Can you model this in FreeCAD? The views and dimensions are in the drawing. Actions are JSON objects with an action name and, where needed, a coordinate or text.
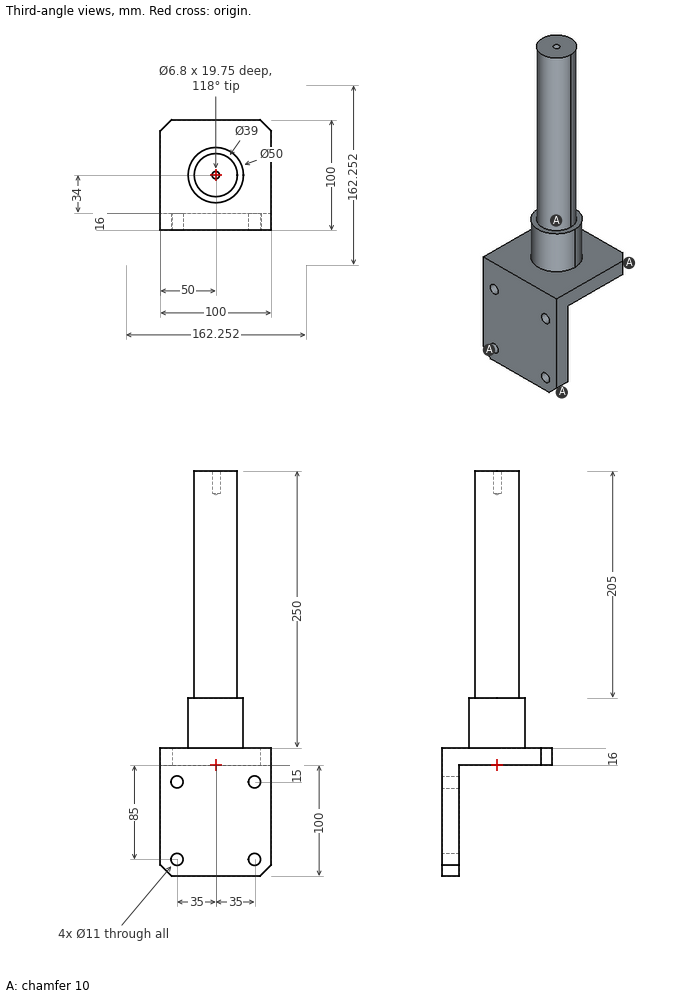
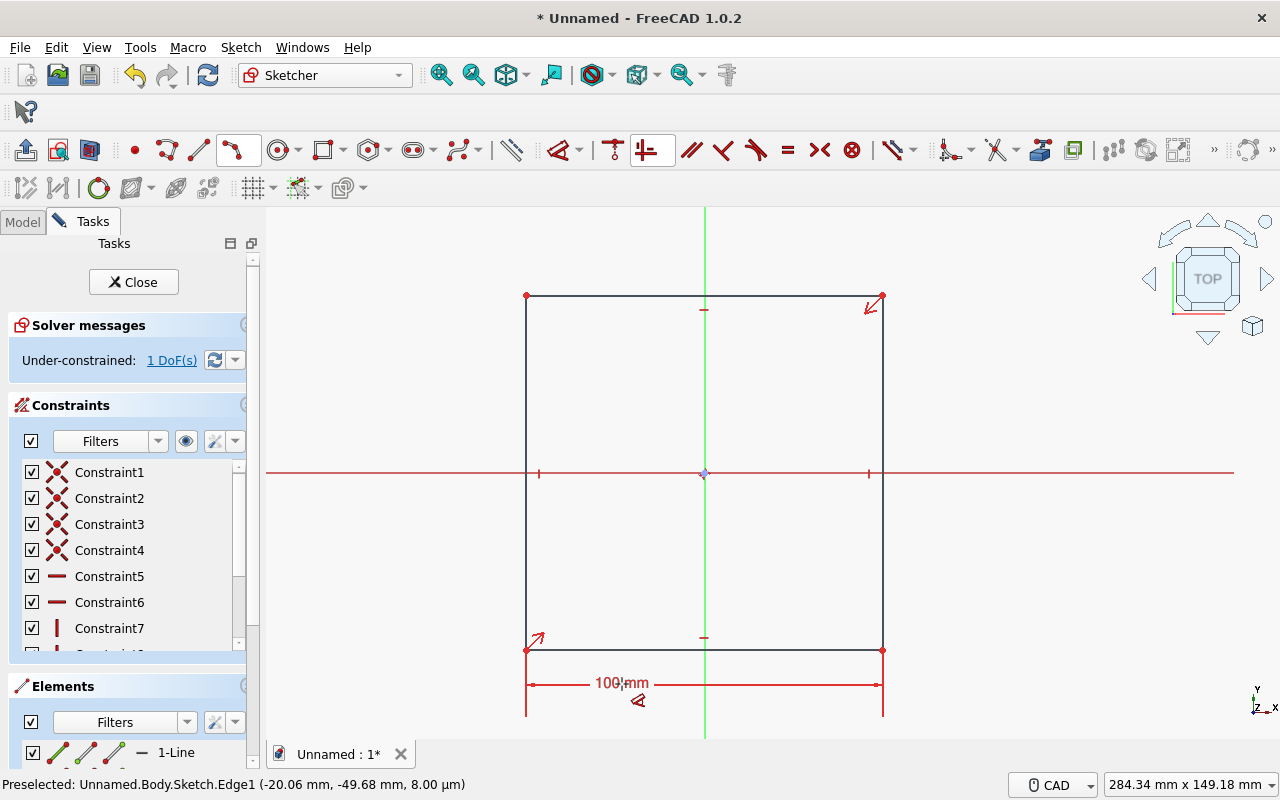
{"action": "left_click", "coordinate": [883, 544]}
{"action": "left_click", "coordinate": [917, 392]}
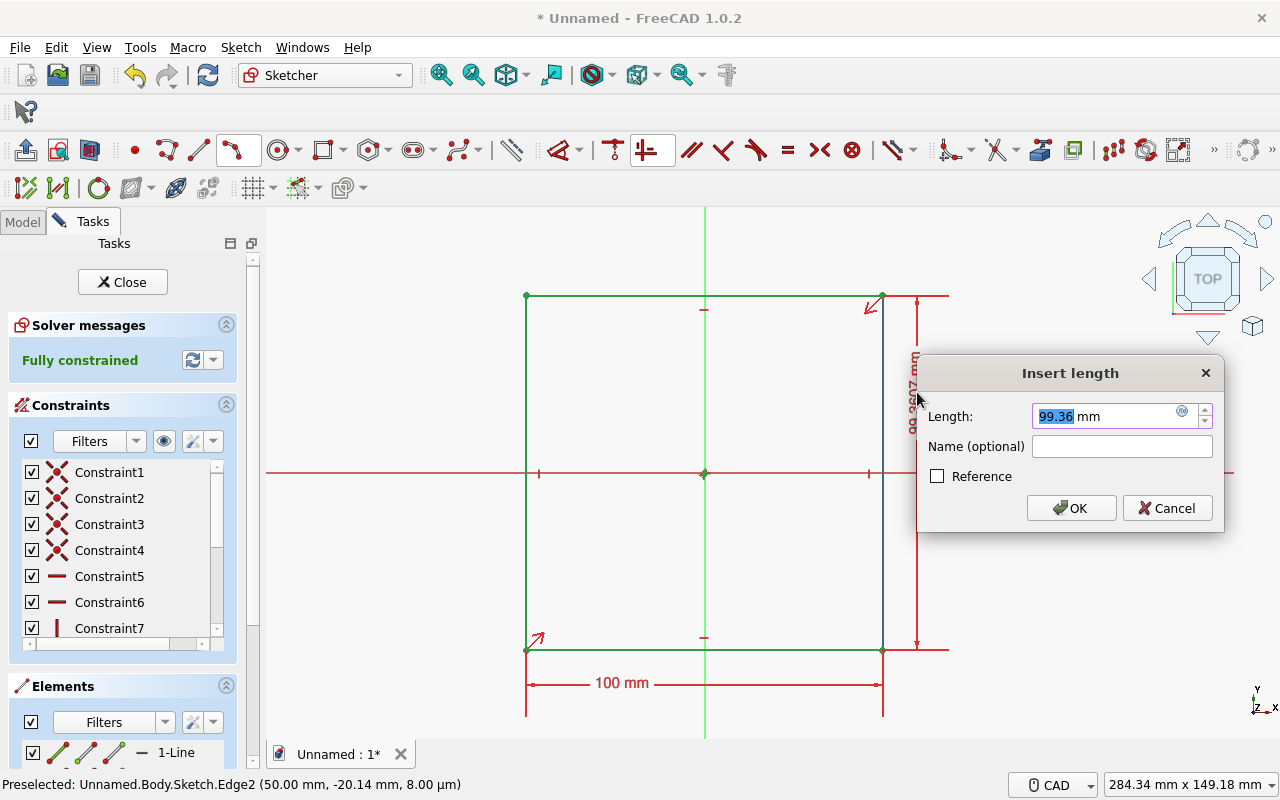
{"action": "type", "text": "100"}
{"action": "key", "text": "Return"}
{"action": "key", "text": "Escape"}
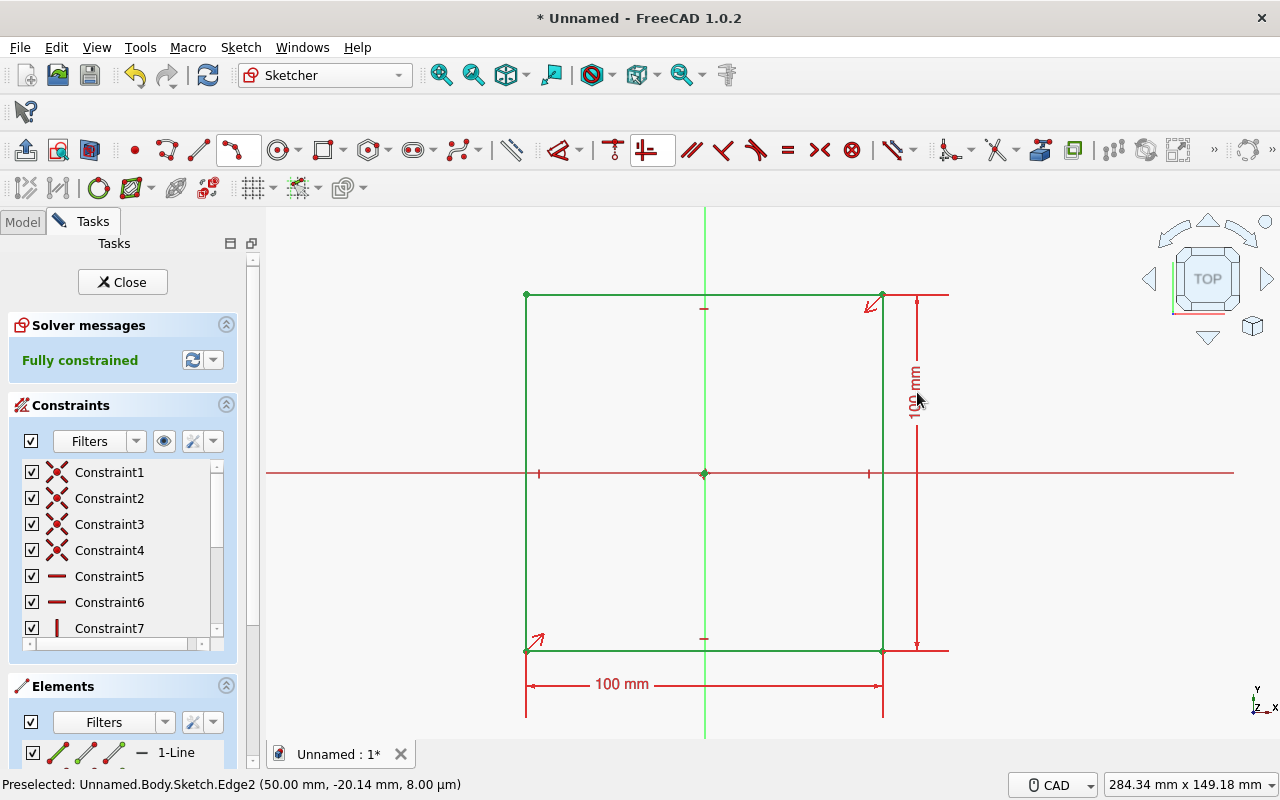
{"action": "left_click", "coordinate": [123, 282]}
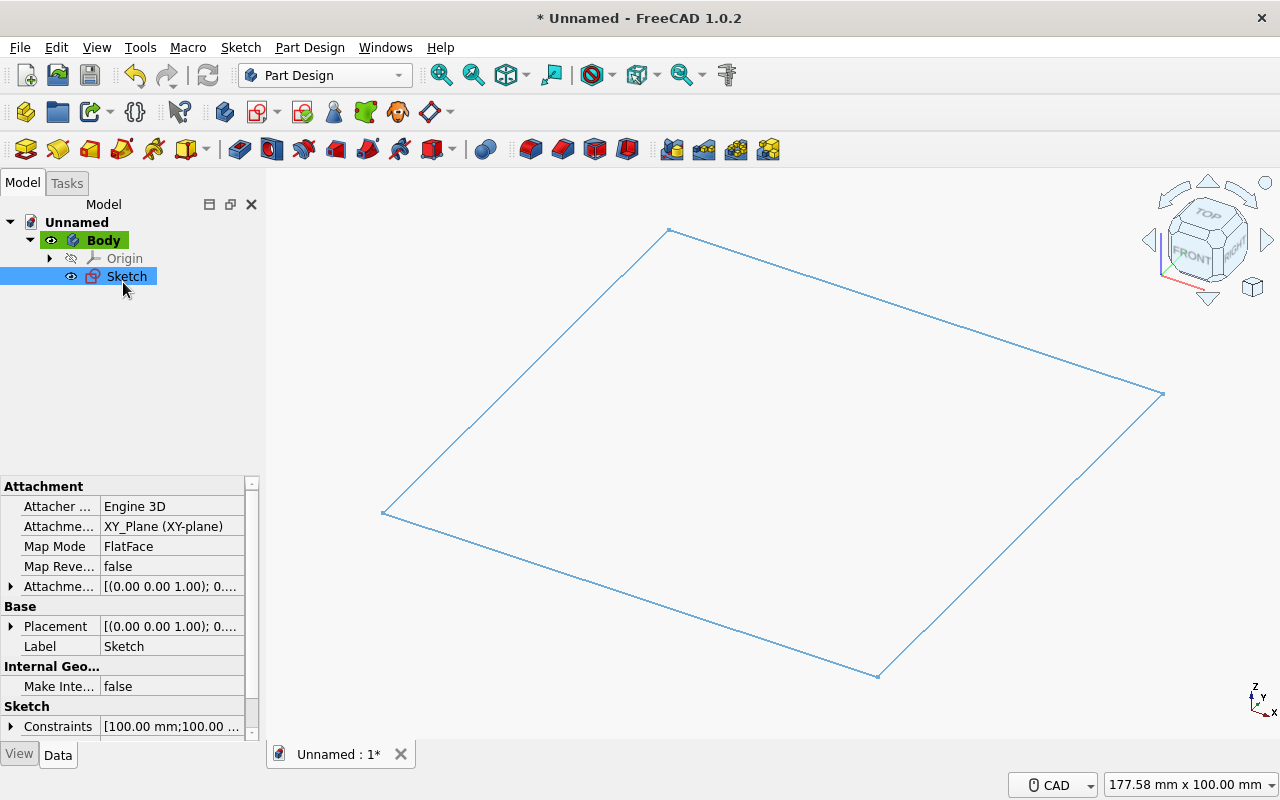
{"action": "left_click", "coordinate": [26, 150]}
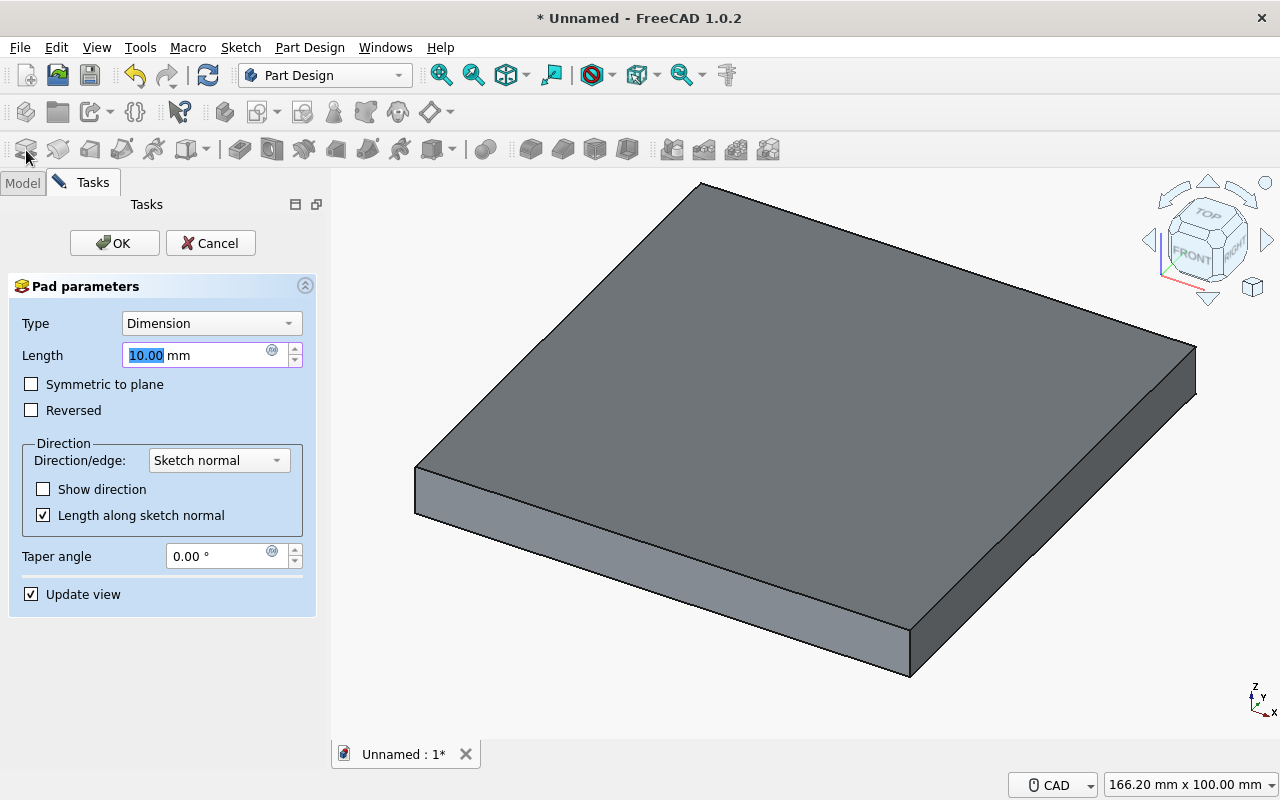
{"action": "type", "text": "16"}
{"action": "key", "text": "Tab"}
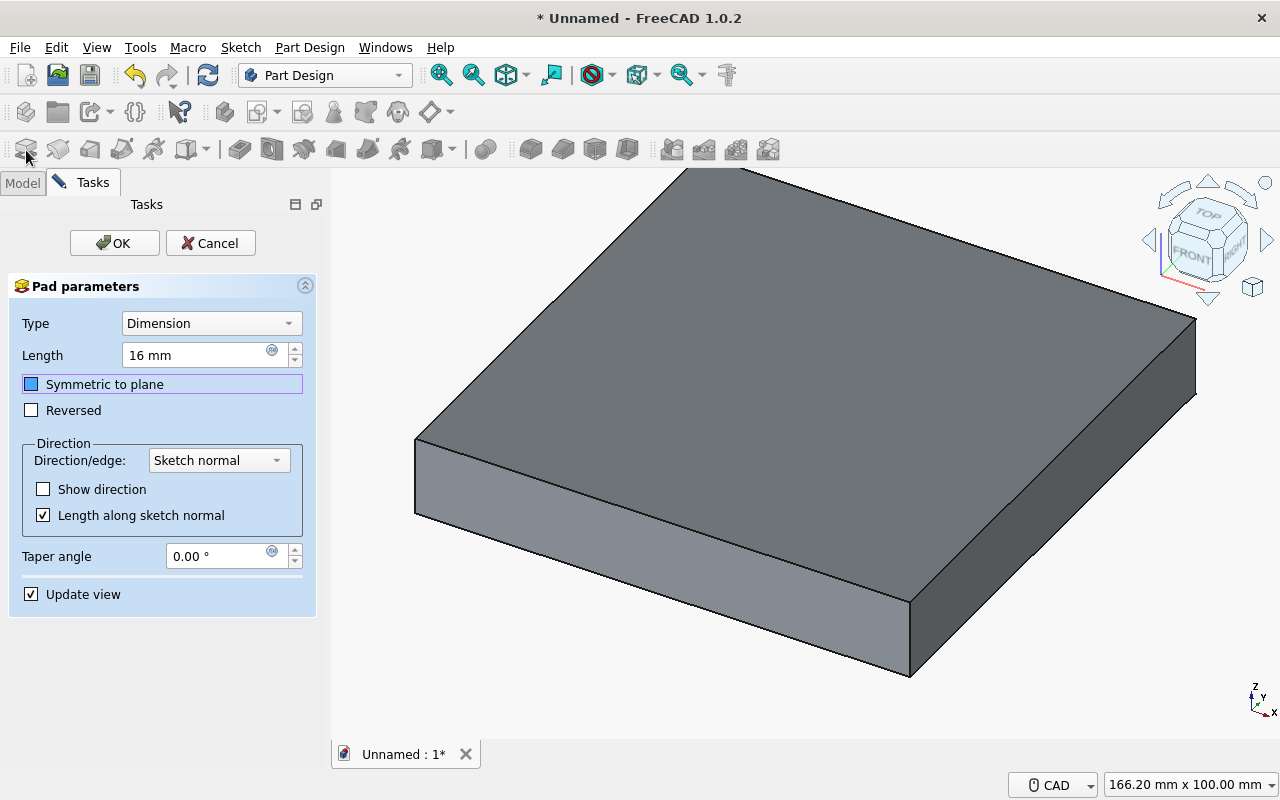
{"action": "left_click", "coordinate": [115, 243]}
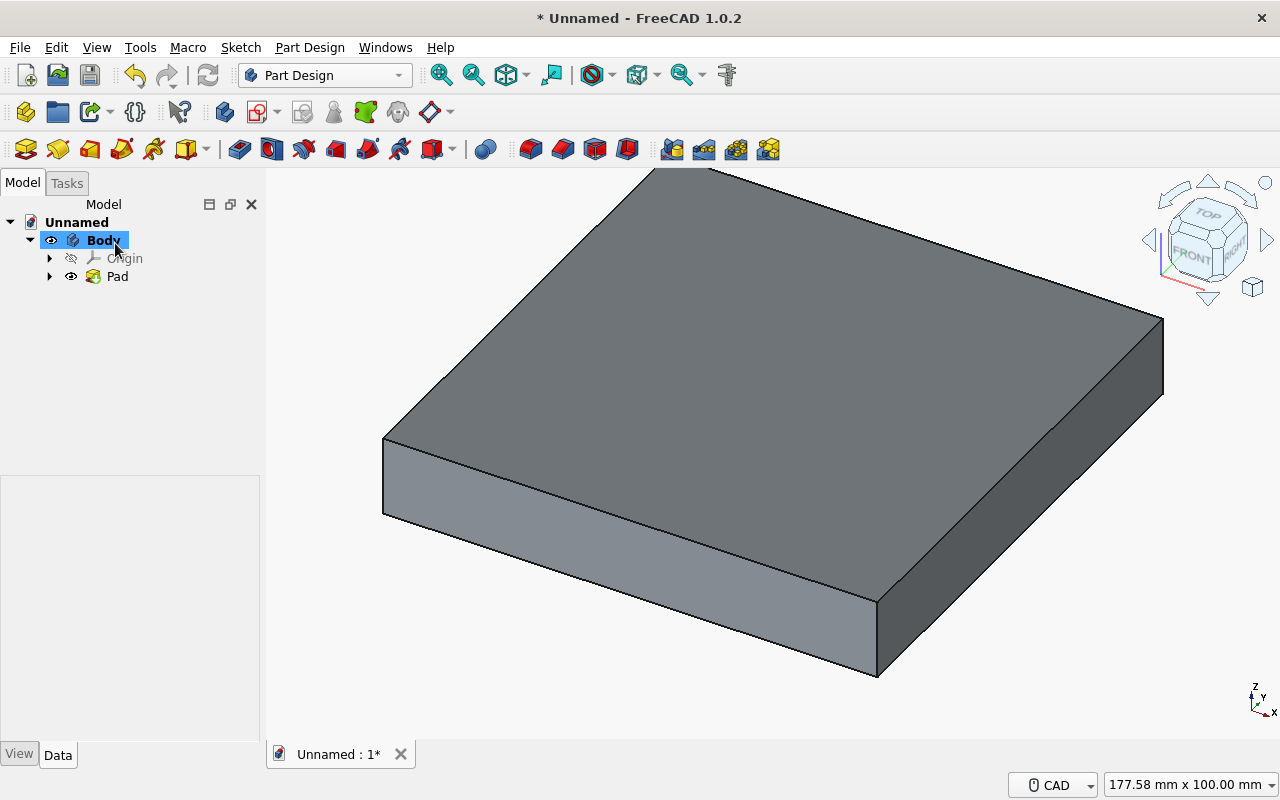
{"action": "left_click", "coordinate": [442, 76]}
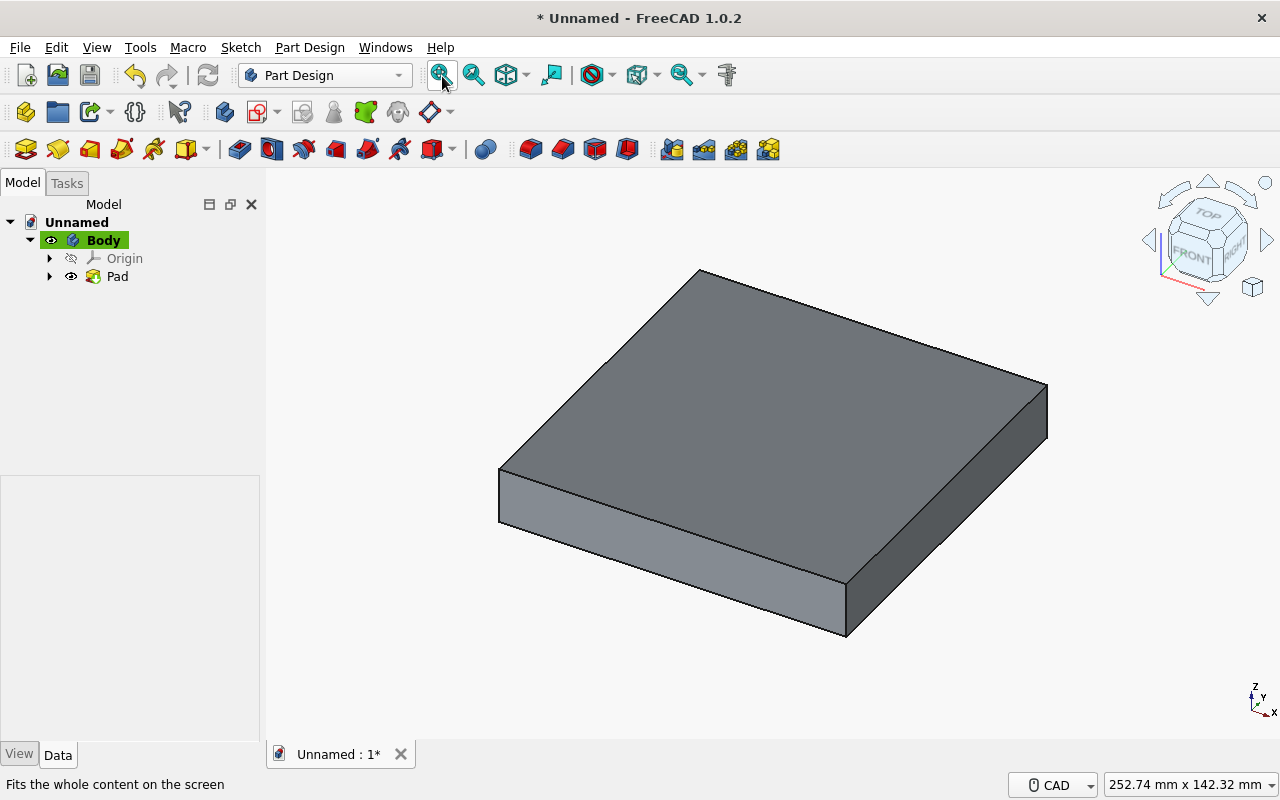
{"action": "left_click", "coordinate": [773, 426]}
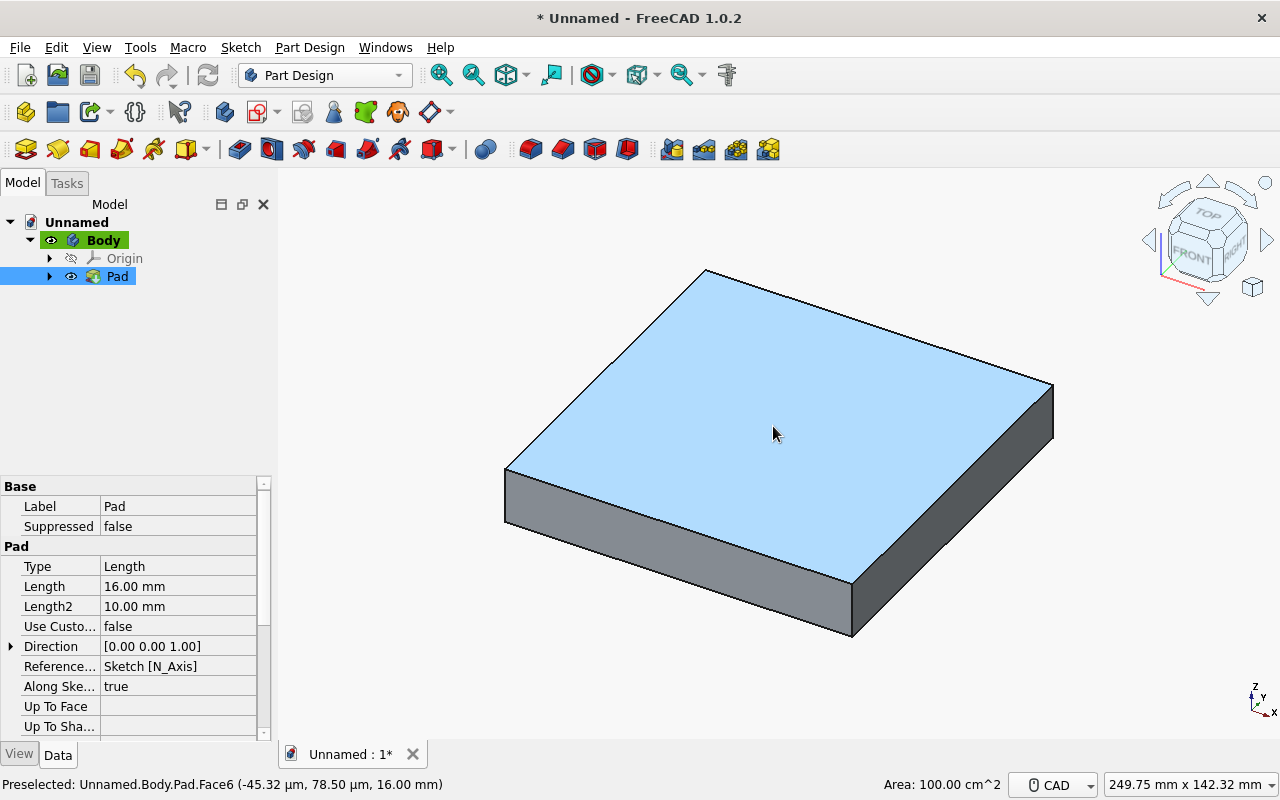
{"action": "left_click", "coordinate": [258, 112]}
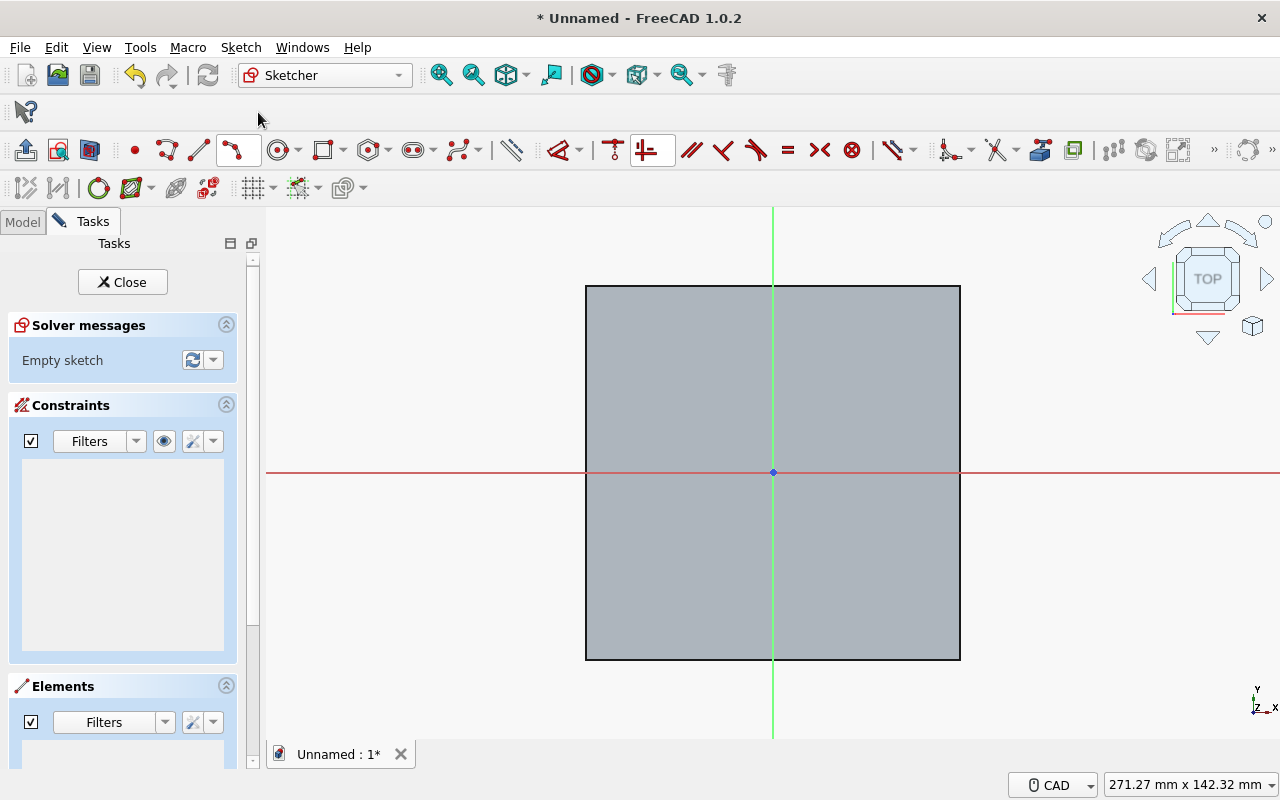
{"action": "scroll", "coordinate": [856, 473], "scroll_direction": "up", "scroll_amount": 3}